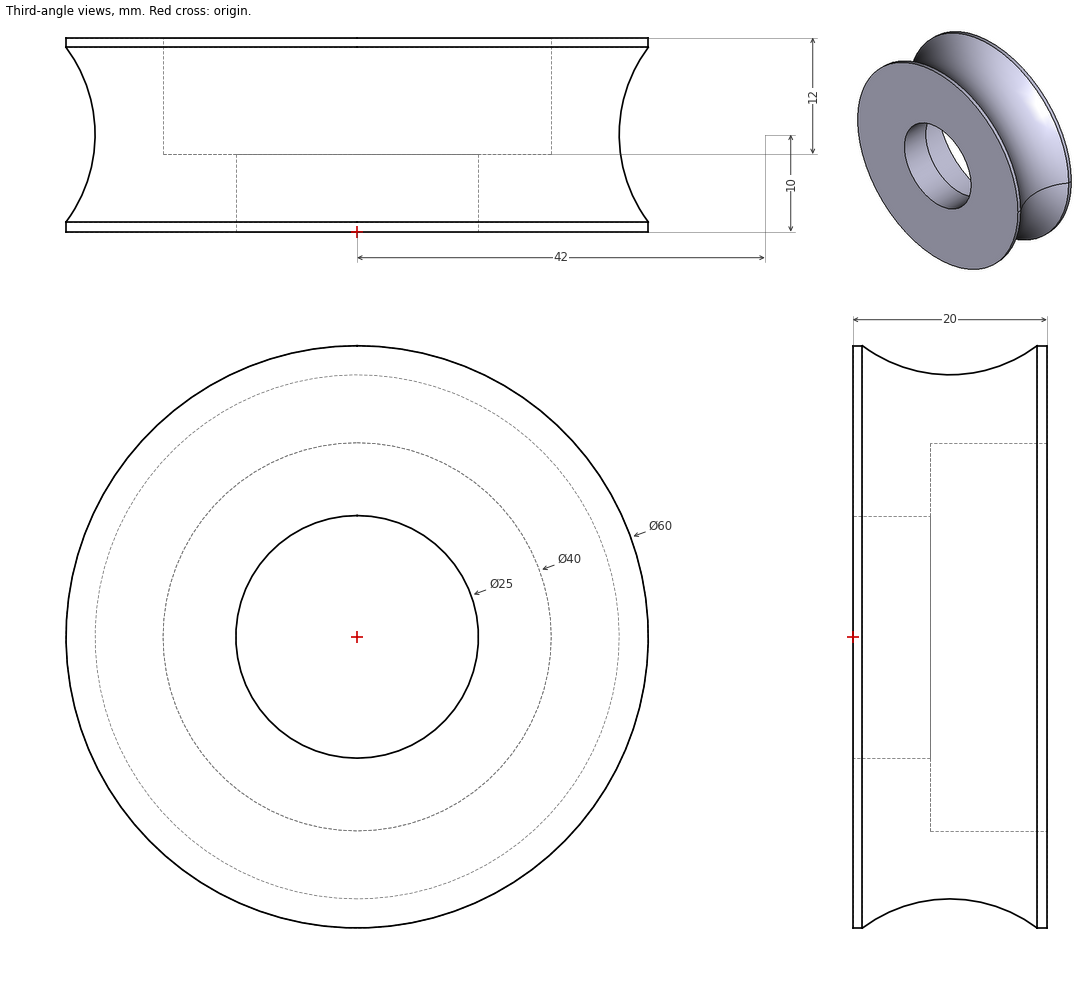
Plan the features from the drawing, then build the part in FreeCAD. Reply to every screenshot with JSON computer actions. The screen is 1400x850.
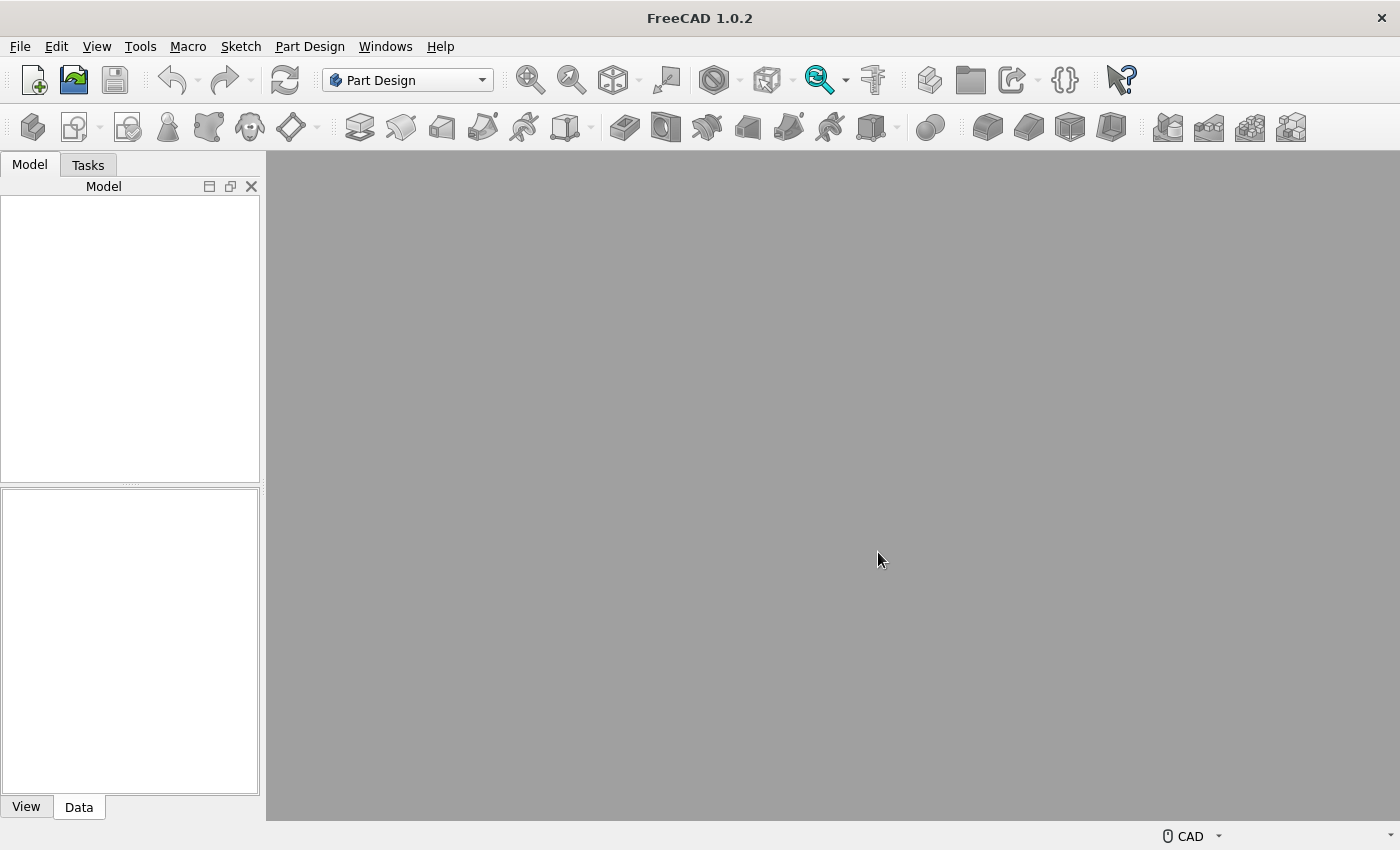
{"action": "left_click", "coordinate": [33, 80]}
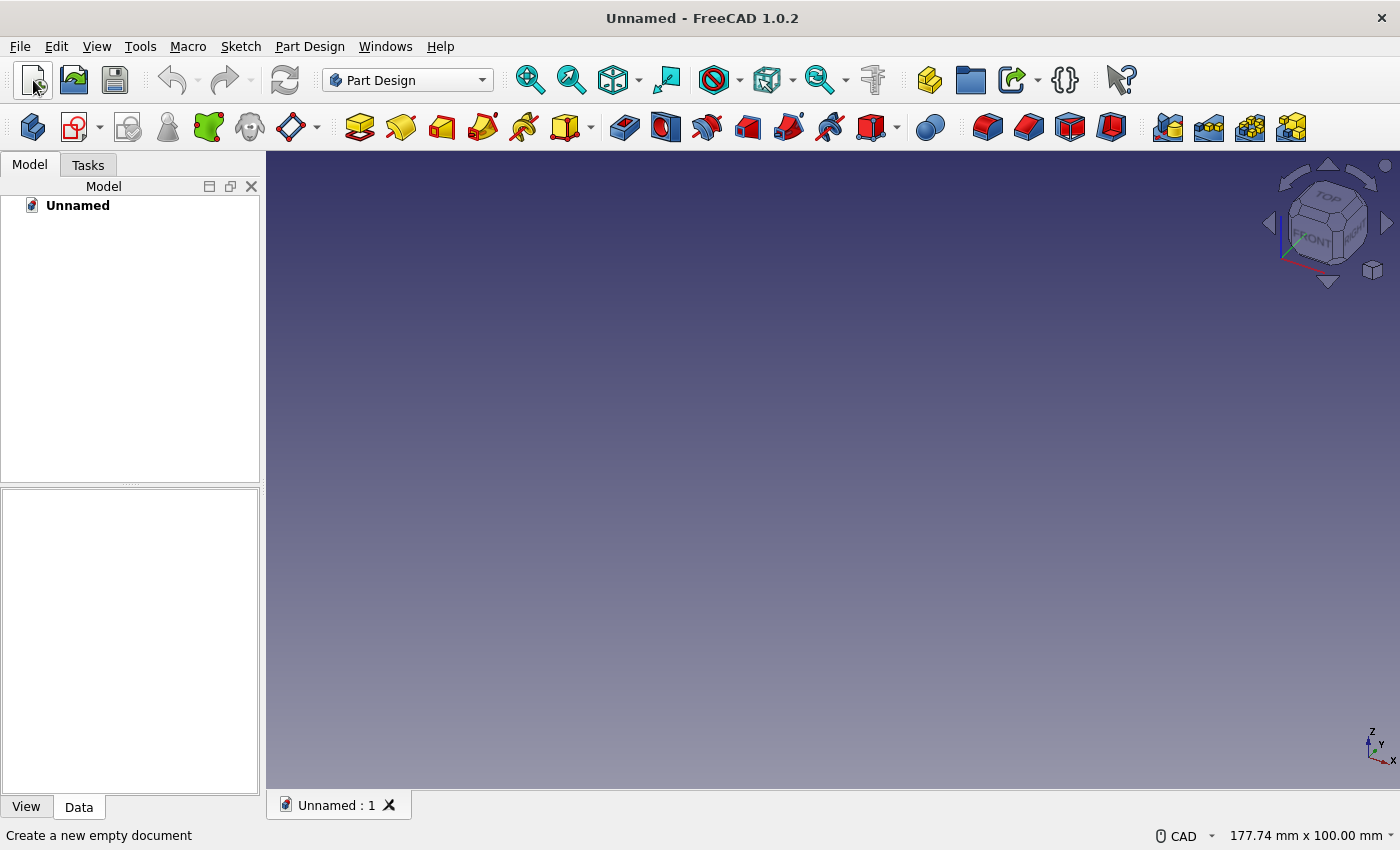
{"action": "left_click", "coordinate": [74, 128]}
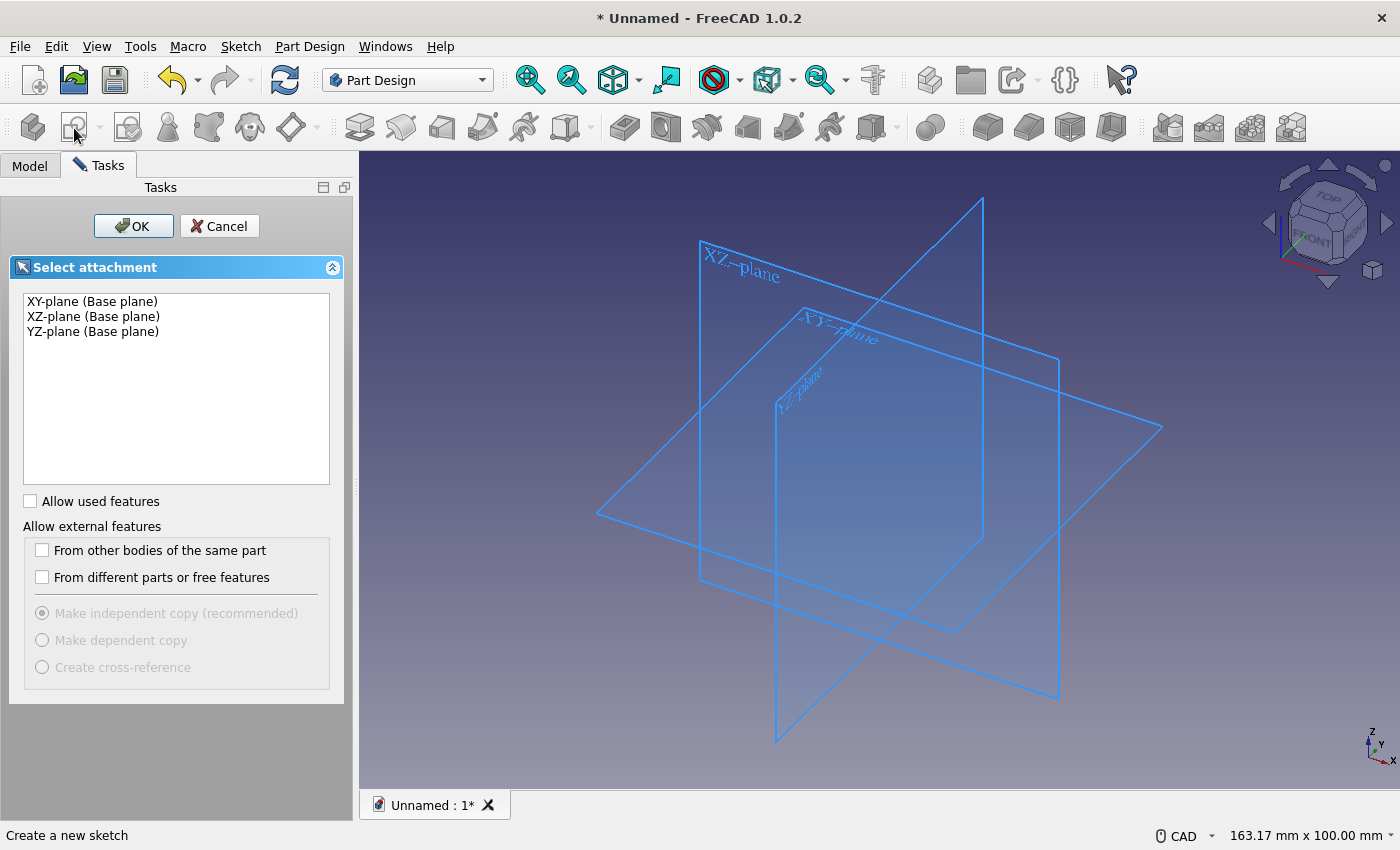
{"action": "left_click", "coordinate": [84, 316]}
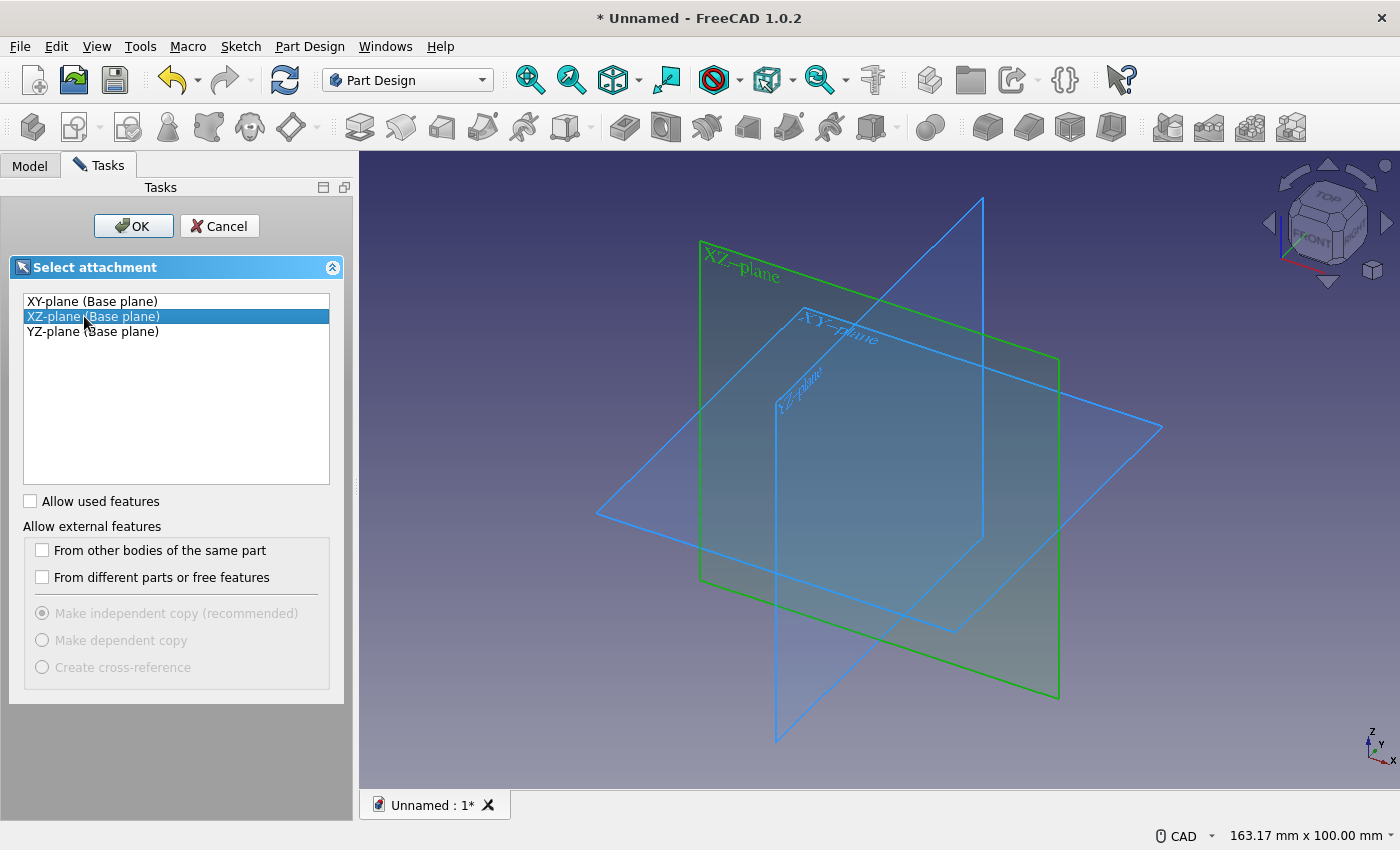
{"action": "left_click", "coordinate": [134, 226]}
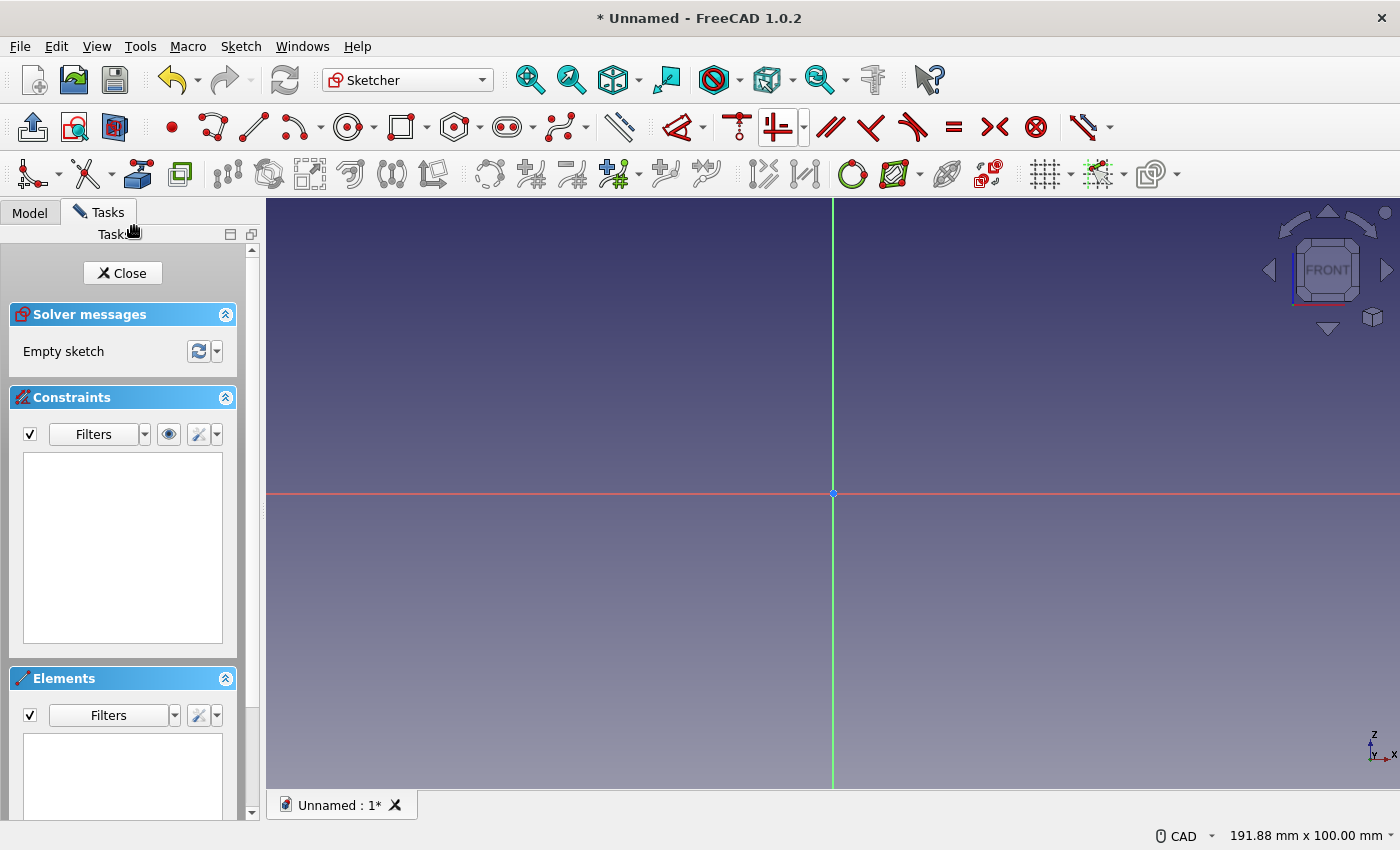
{"action": "left_click", "coordinate": [348, 128]}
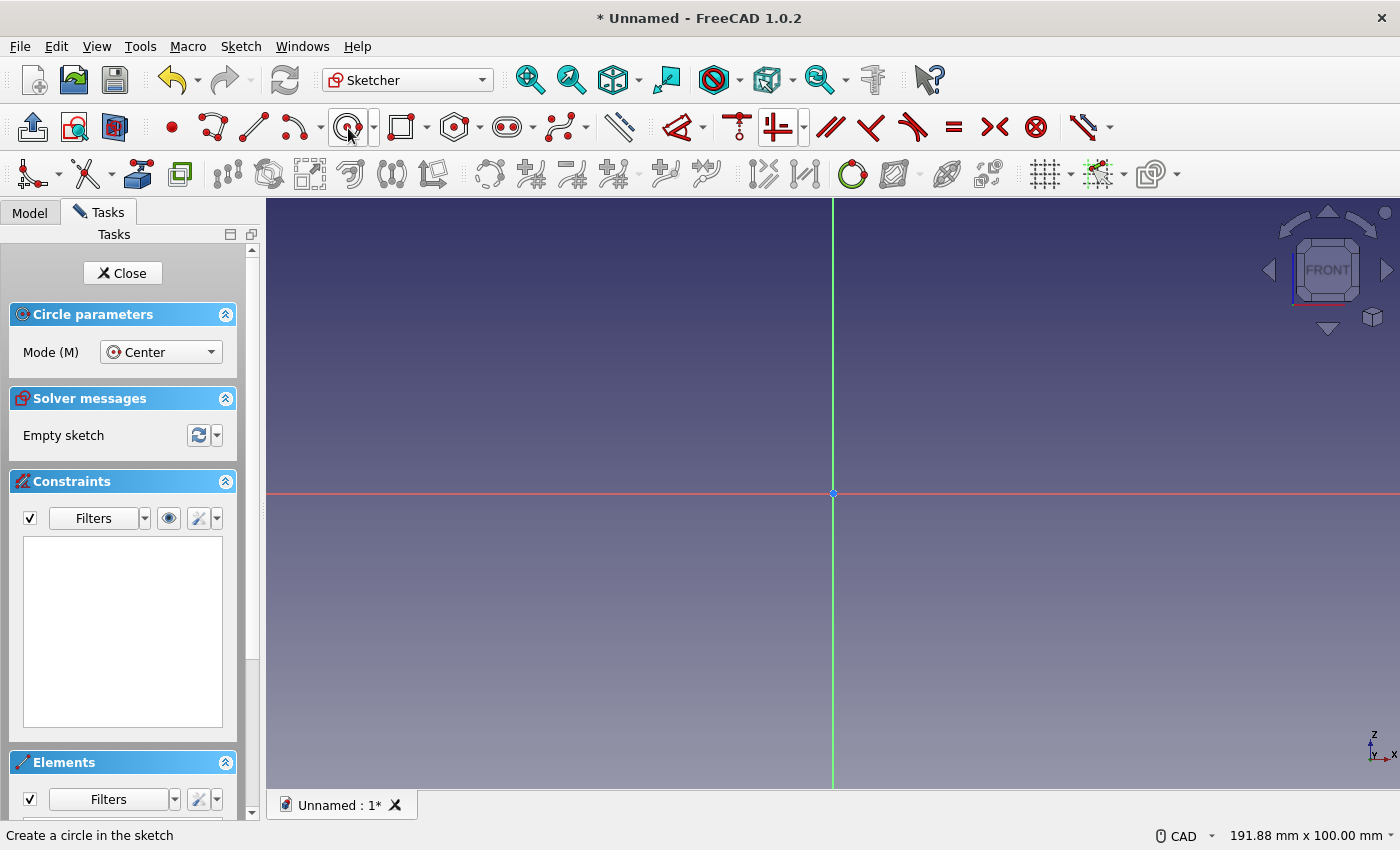
{"action": "left_click", "coordinate": [833, 494]}
{"action": "left_click", "coordinate": [958, 368]}
{"action": "key", "text": "Escape"}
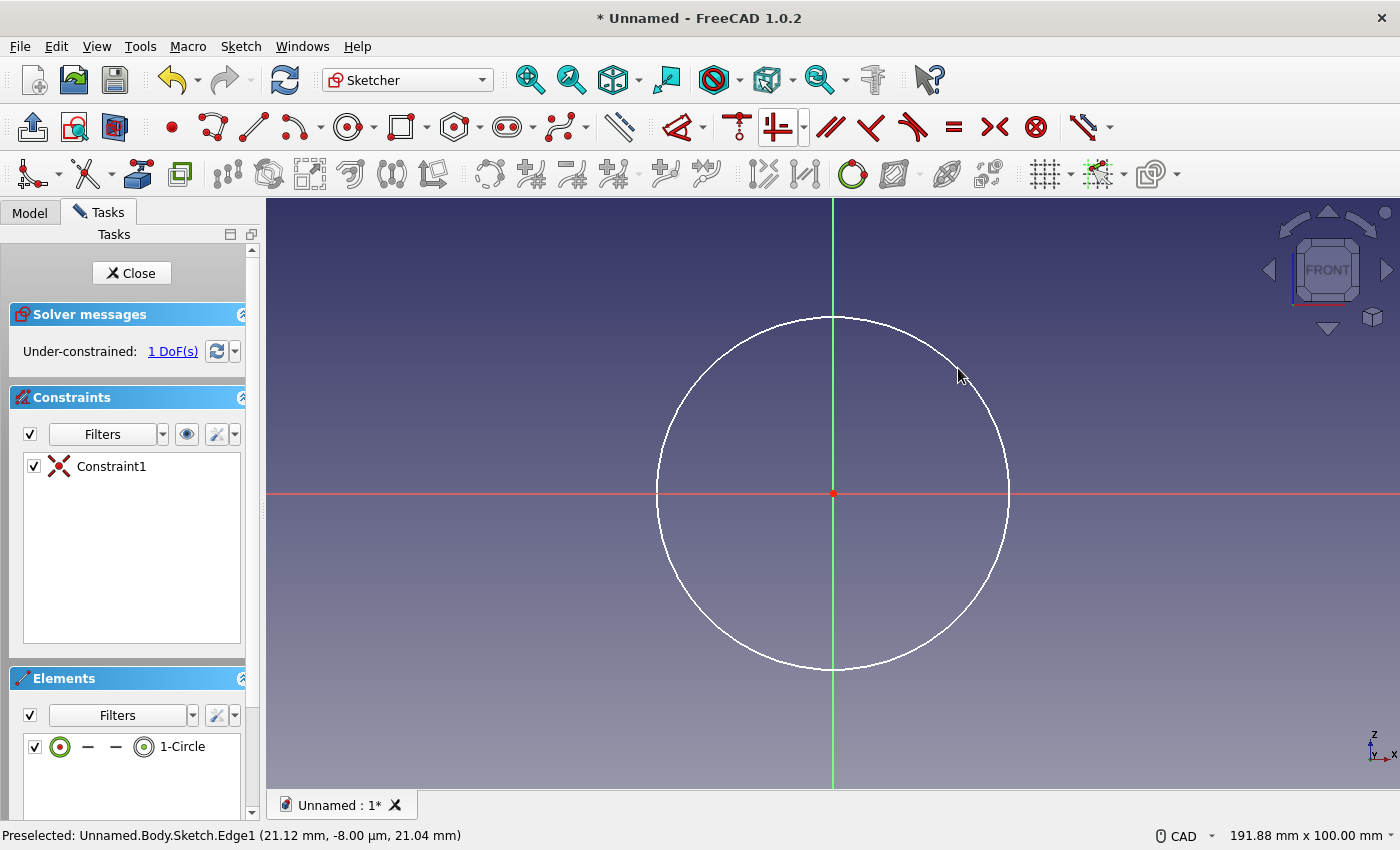
{"action": "left_click", "coordinate": [676, 128]}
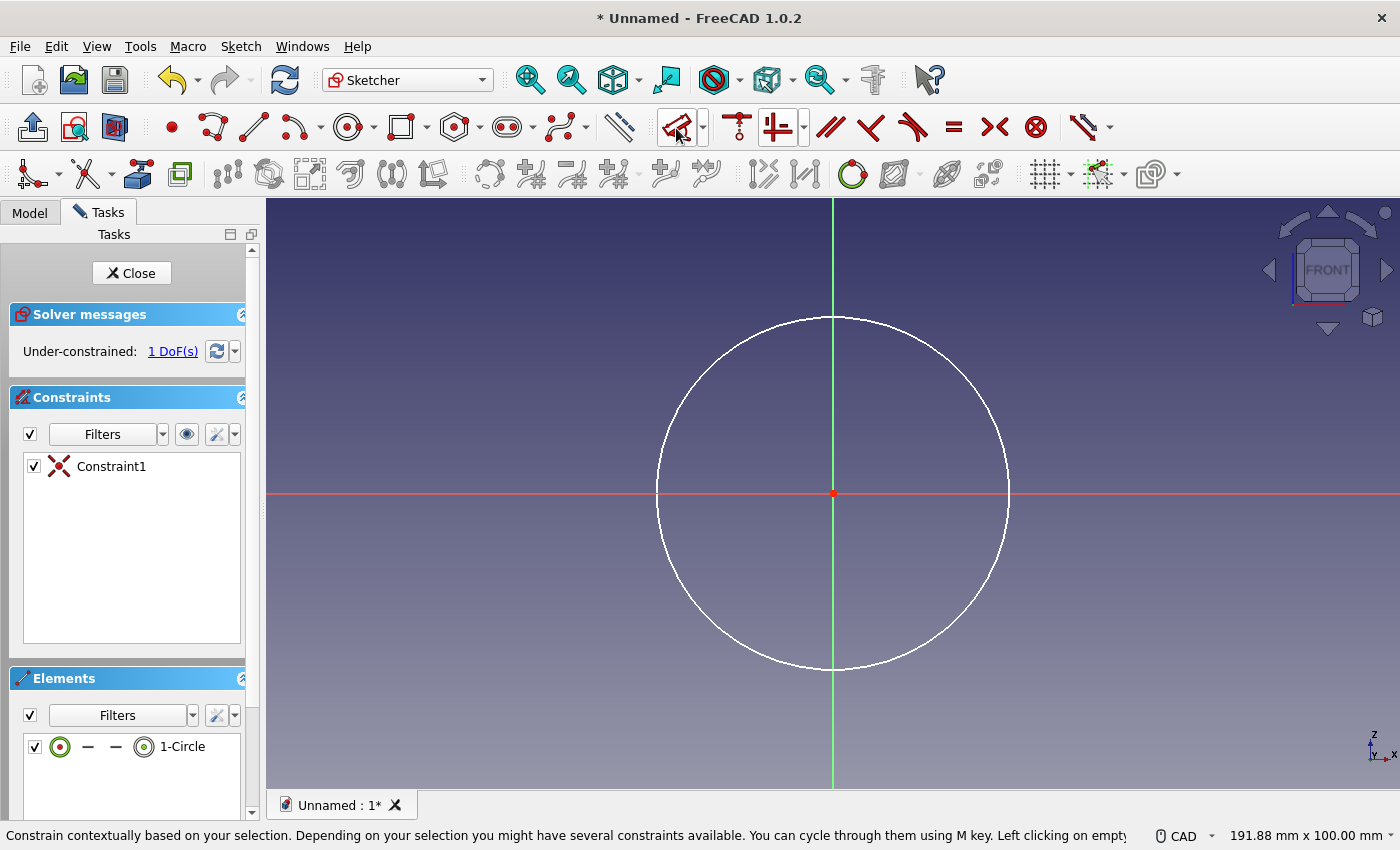
{"action": "left_click", "coordinate": [957, 368]}
{"action": "left_click", "coordinate": [979, 345]}